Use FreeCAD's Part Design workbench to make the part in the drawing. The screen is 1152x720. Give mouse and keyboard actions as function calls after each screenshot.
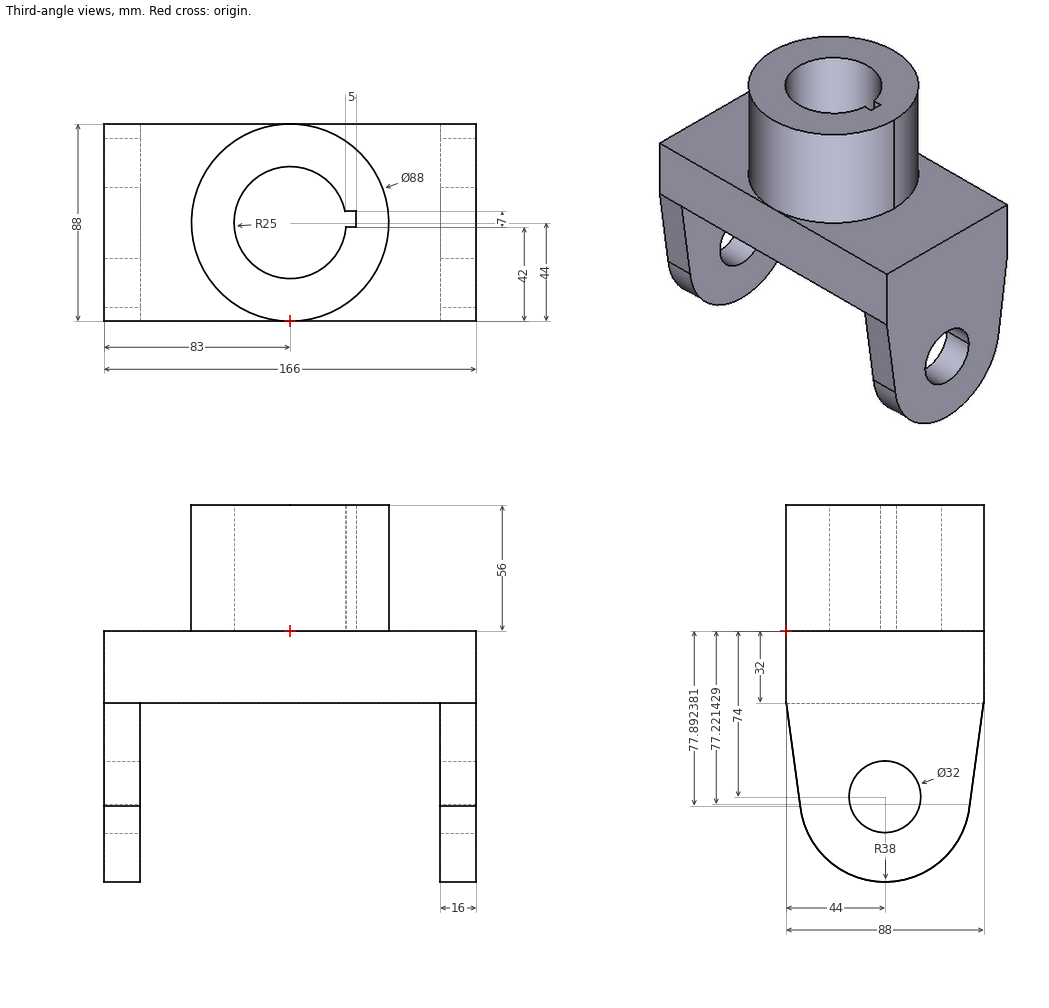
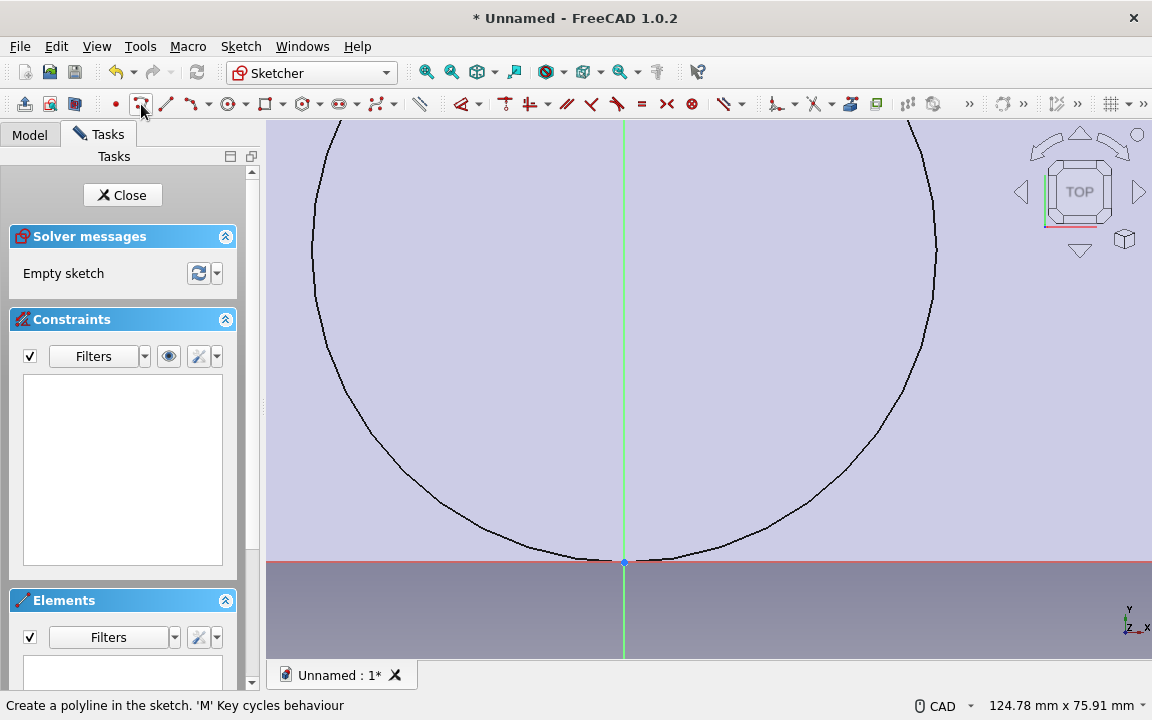
click(801, 264)
click(834, 264)
click(834, 215)
click(798, 215)
right_click(798, 215)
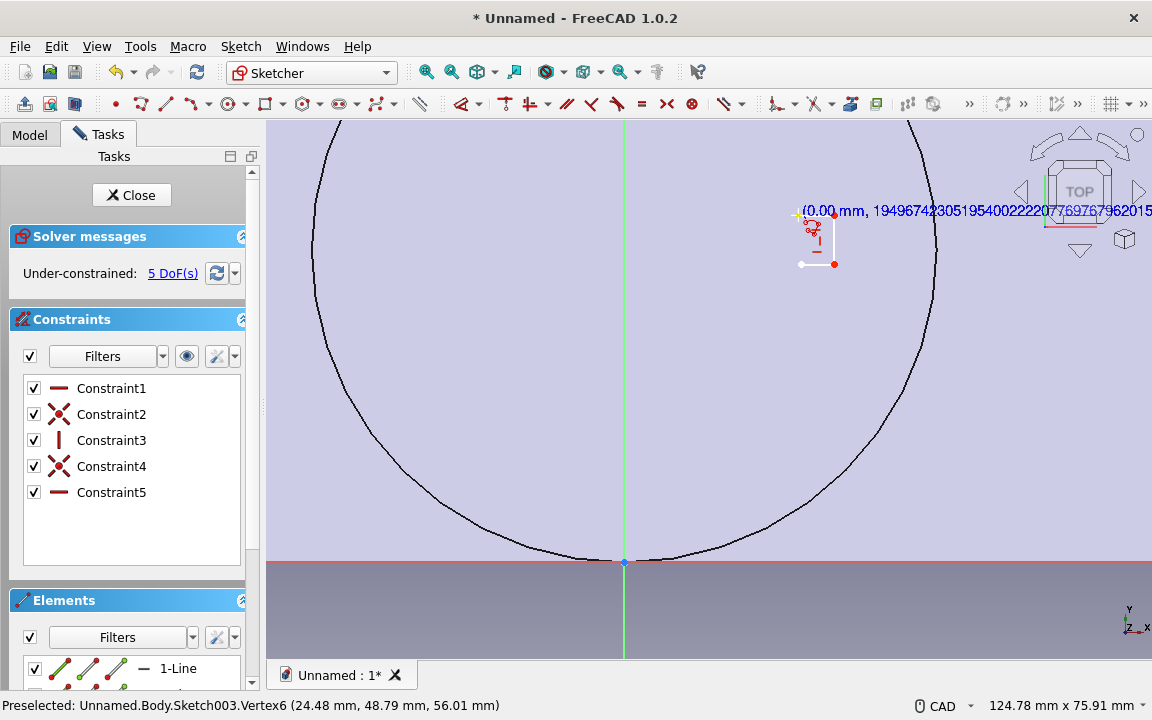
click(190, 104)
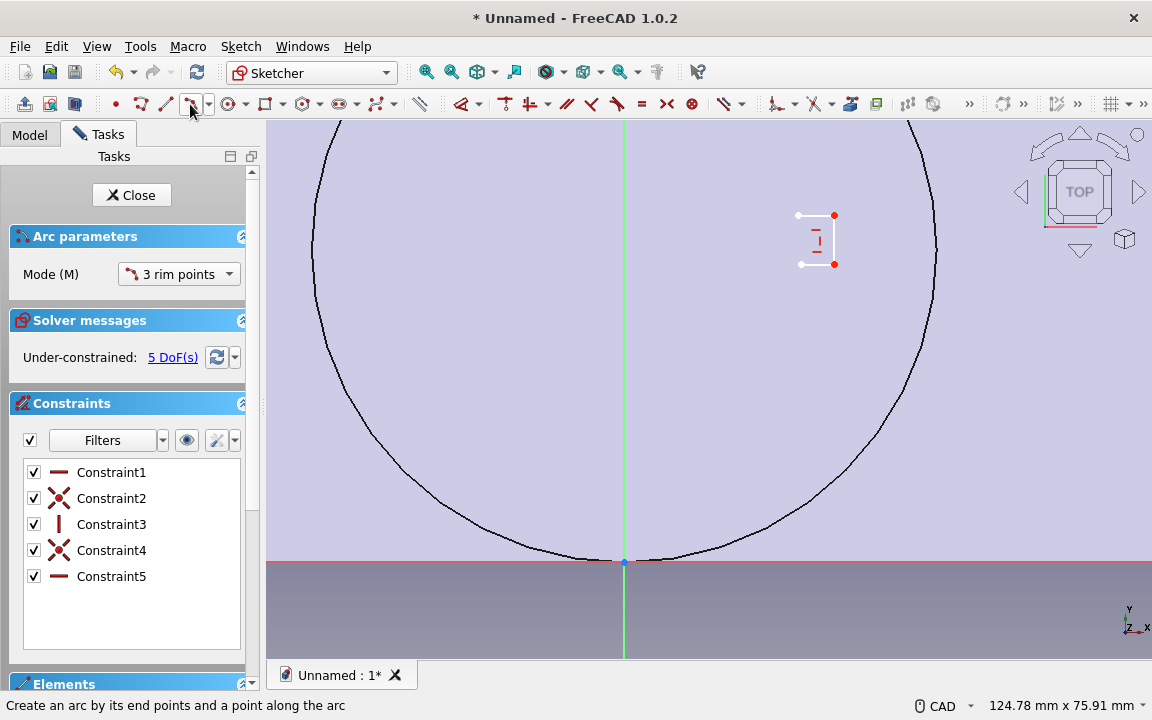
click(798, 216)
click(801, 265)
click(447, 261)
key(Escape)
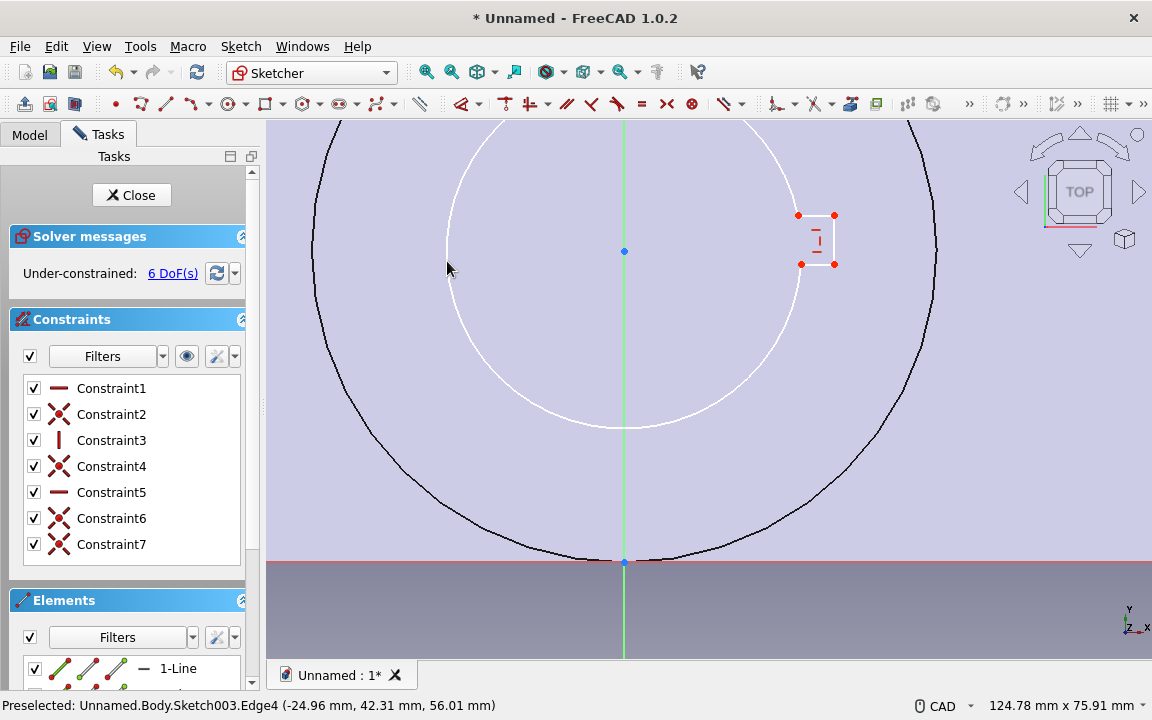
click(624, 251)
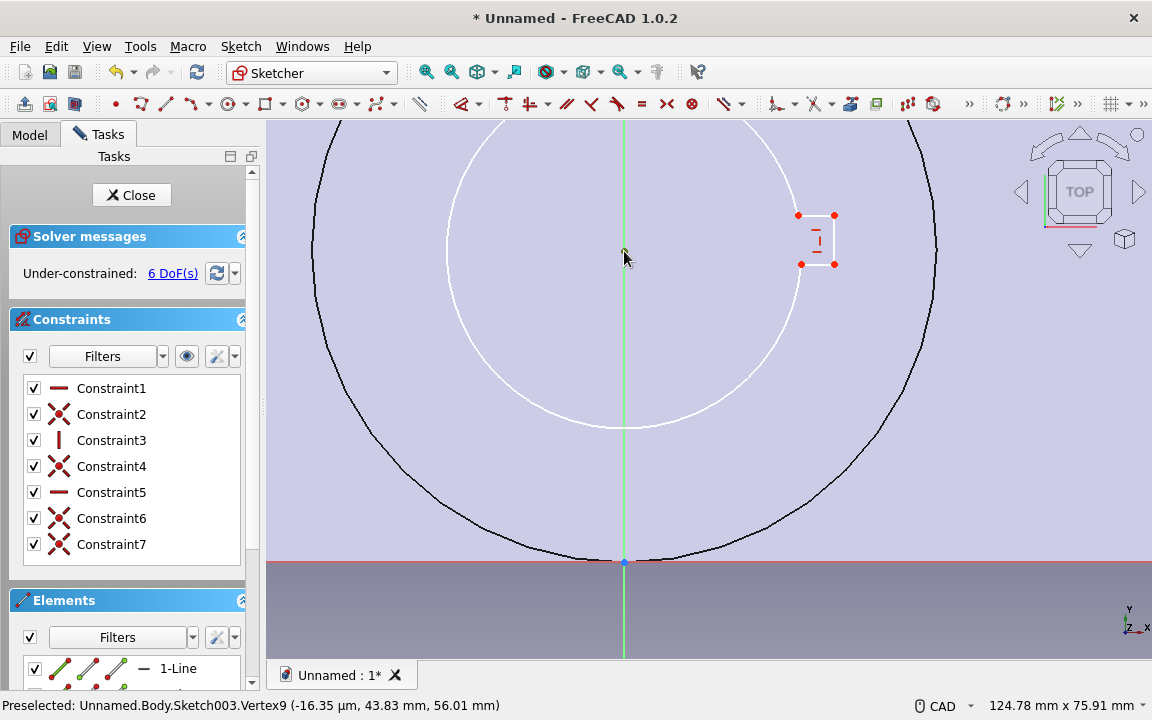
click(624, 596)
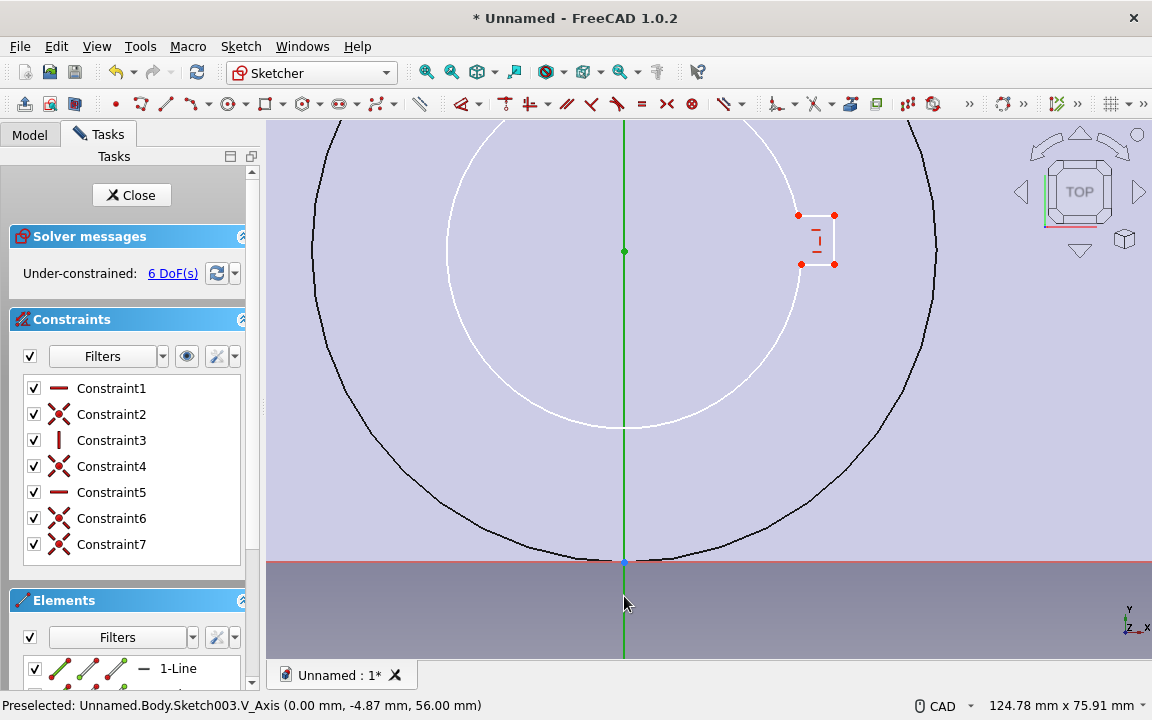
click(505, 104)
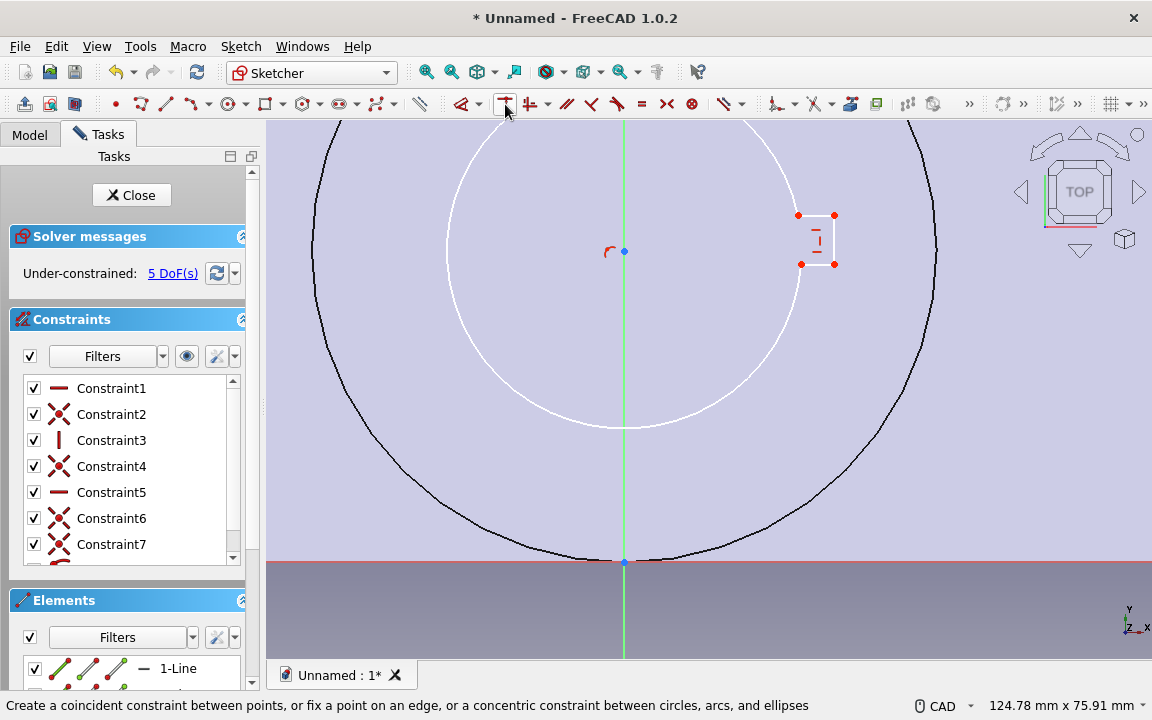
click(460, 104)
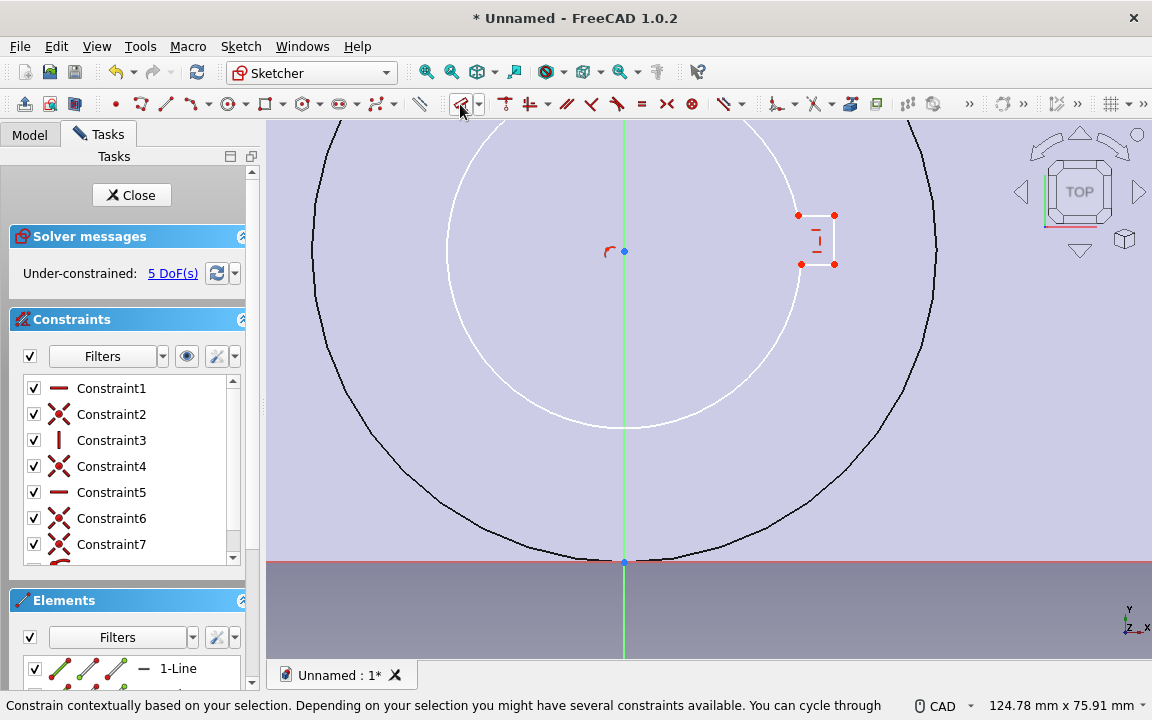
click(570, 420)
click(560, 450)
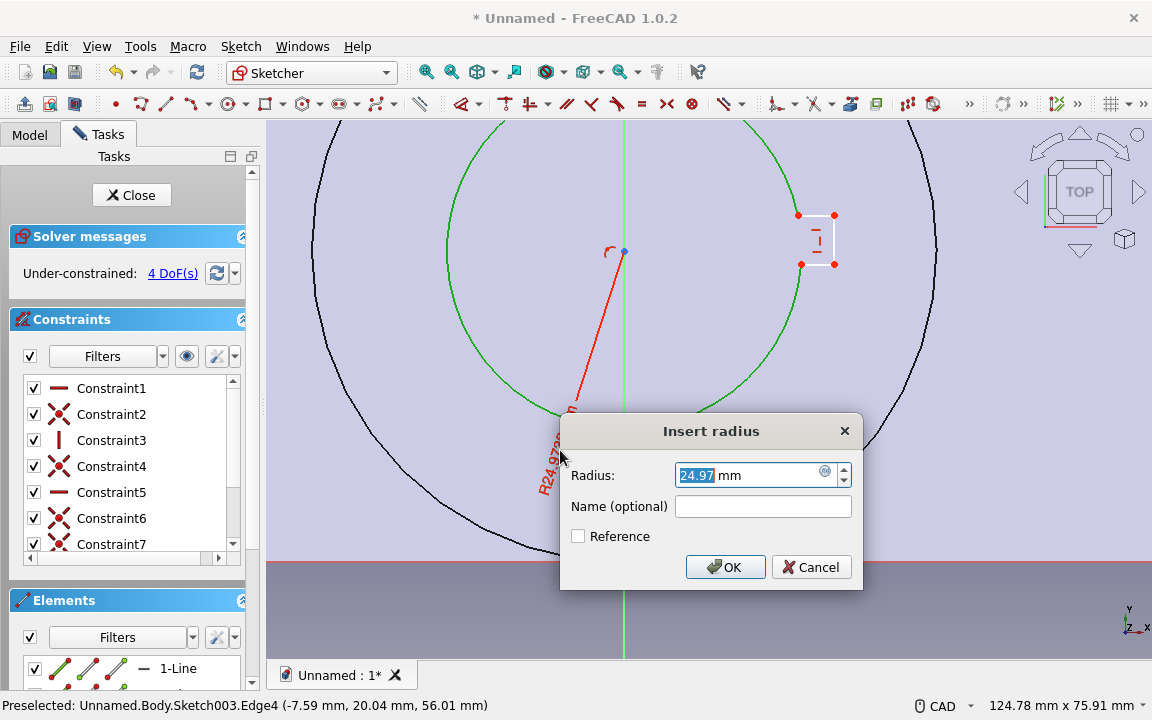
text(25)
key(Return)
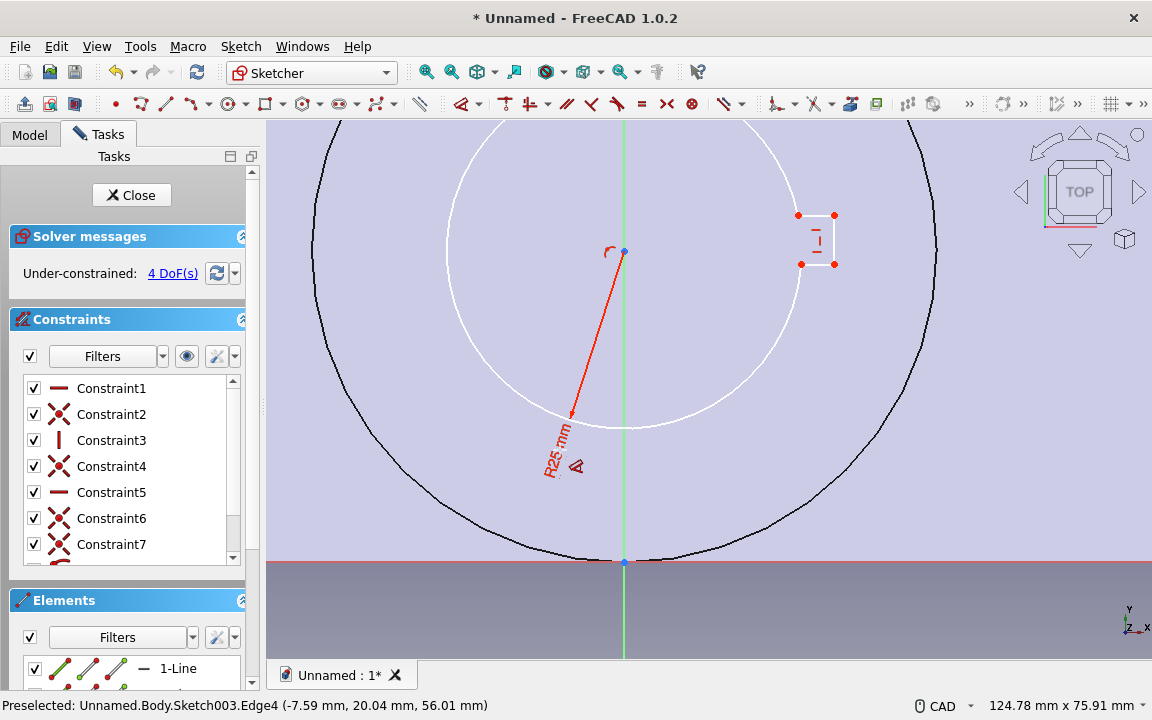
click(834, 250)
click(868, 240)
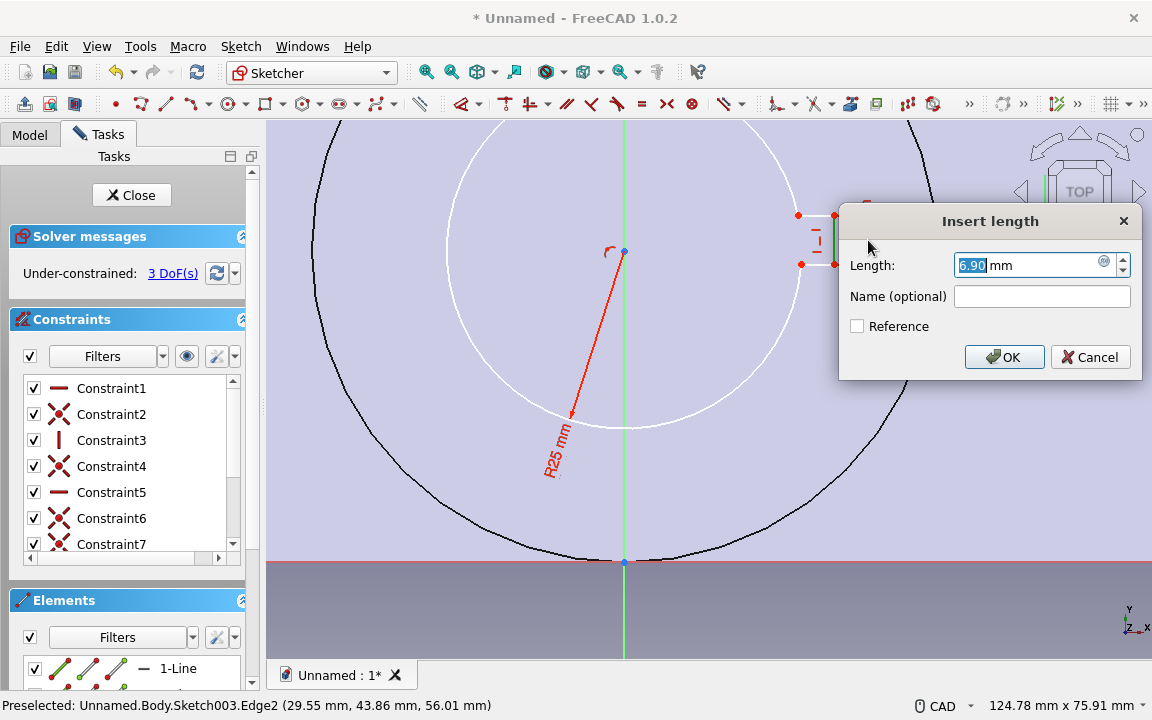
text(7)
key(Return)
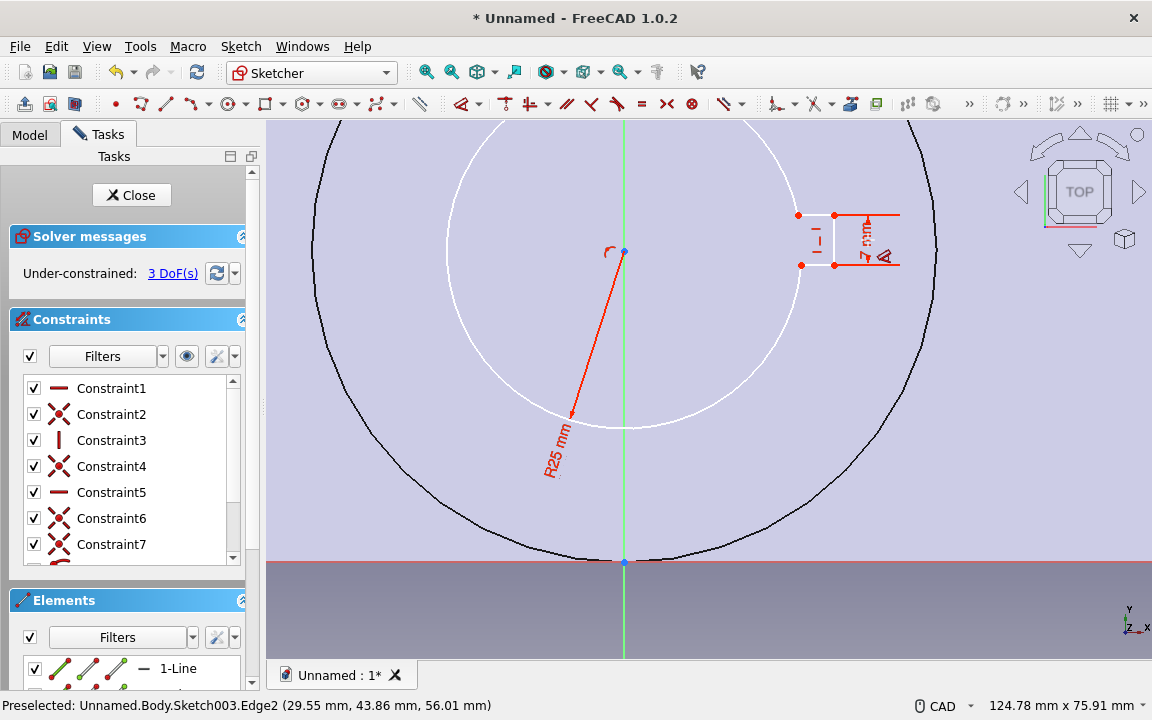
scroll(823, 215, up, 2)